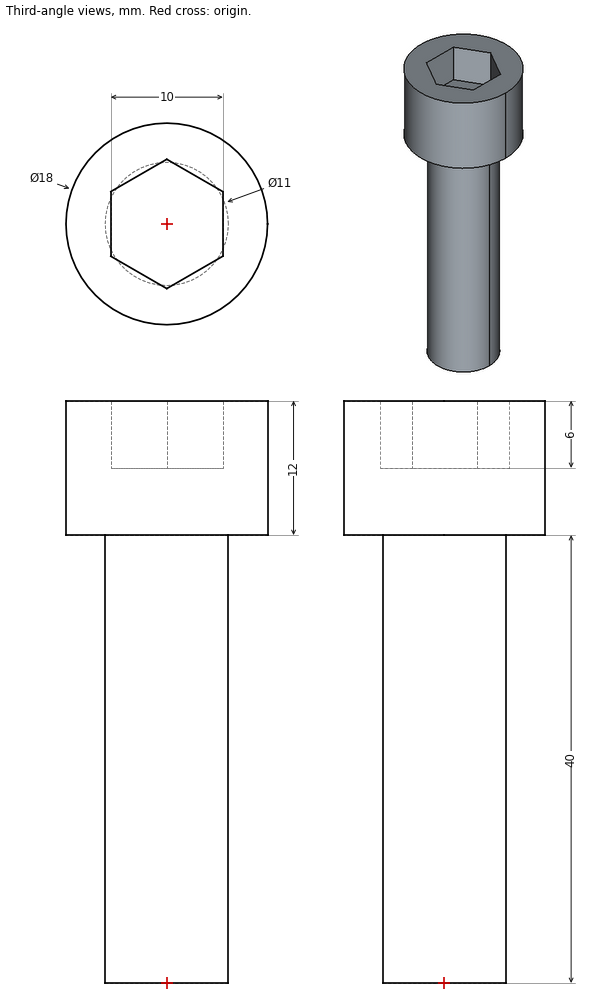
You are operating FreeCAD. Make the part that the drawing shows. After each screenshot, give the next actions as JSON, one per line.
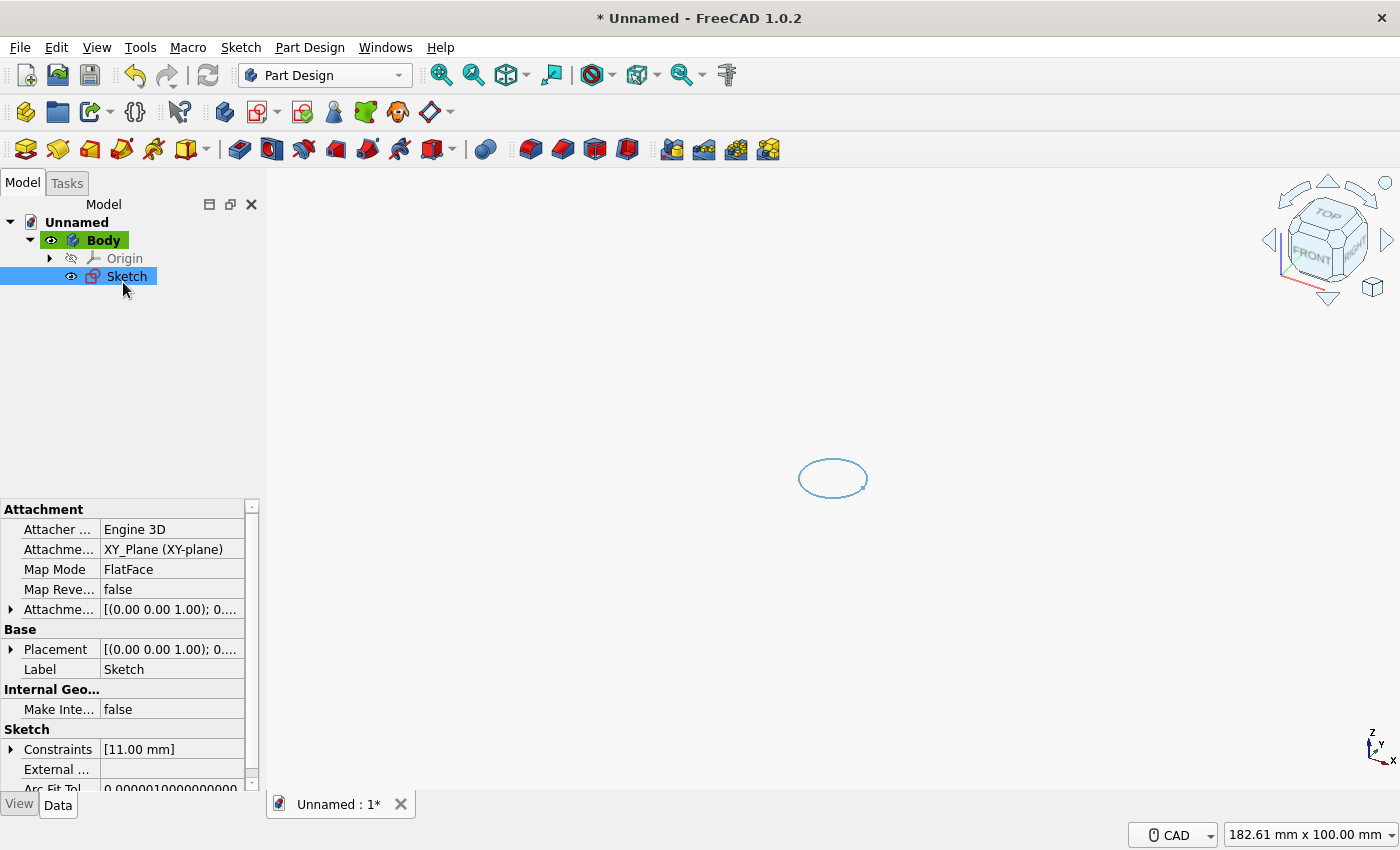
{"action": "left_click", "coordinate": [26, 150]}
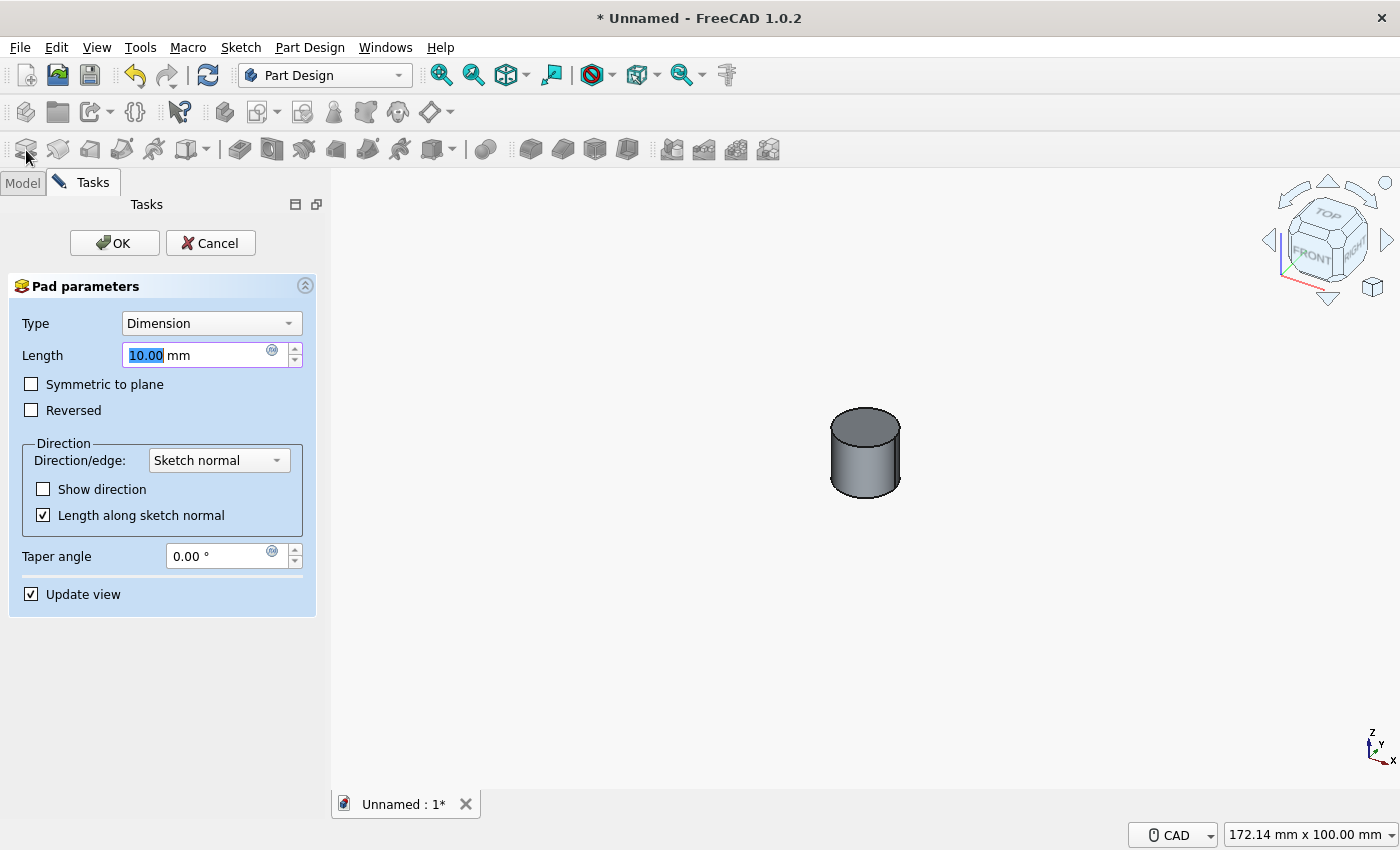
{"action": "type", "text": "40"}
{"action": "key", "text": "Tab"}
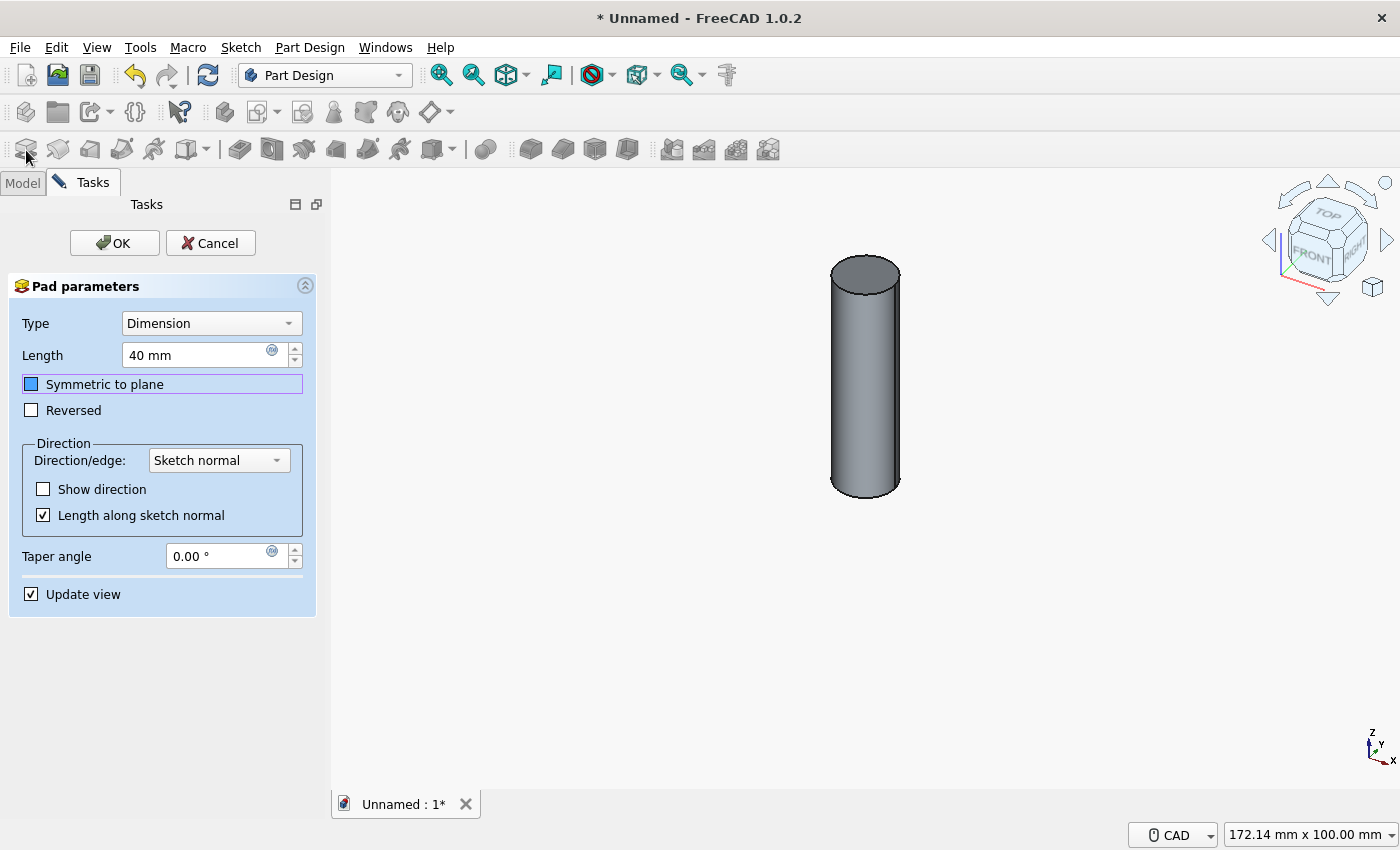
{"action": "left_click", "coordinate": [115, 243]}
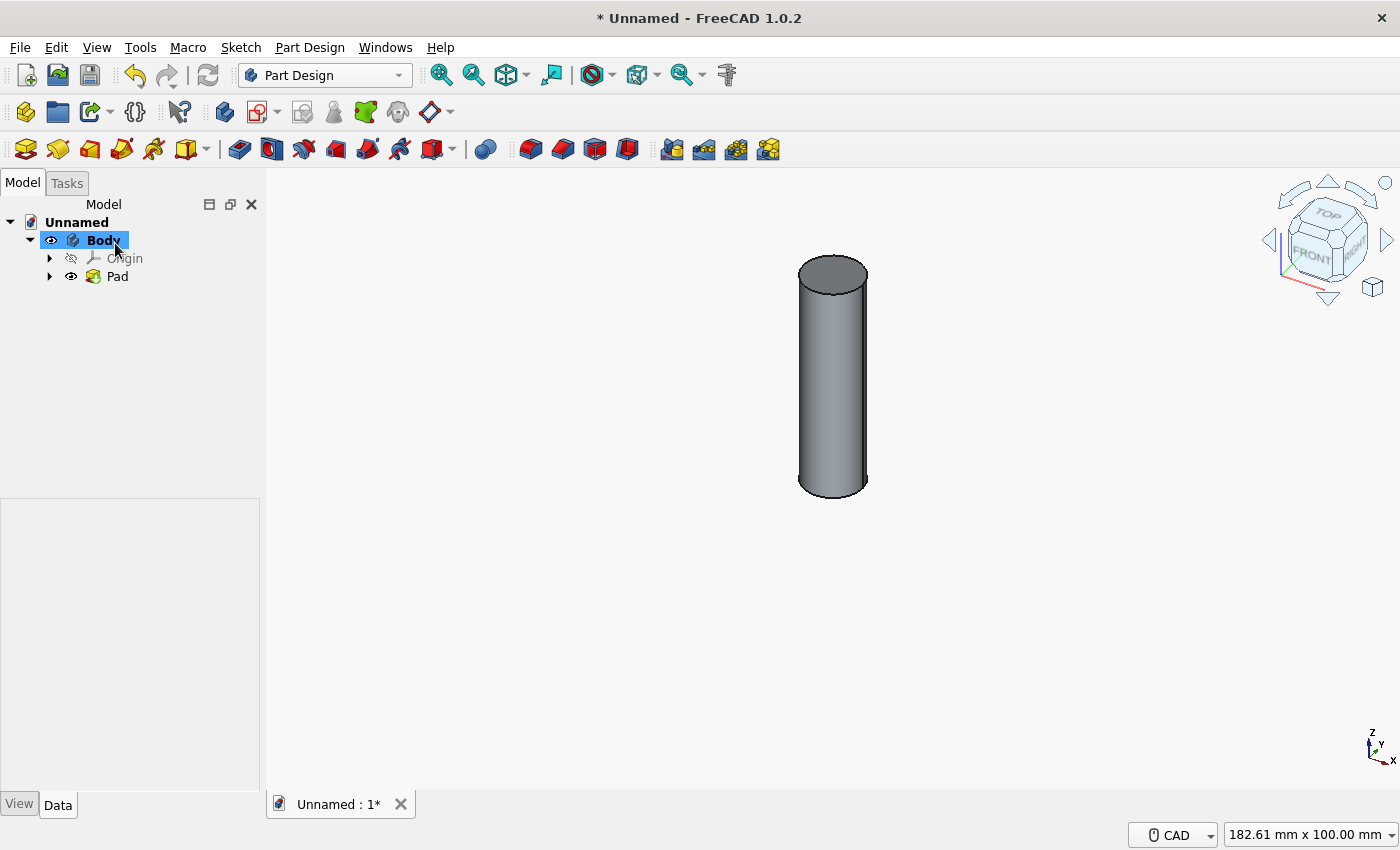
{"action": "left_click", "coordinate": [442, 76]}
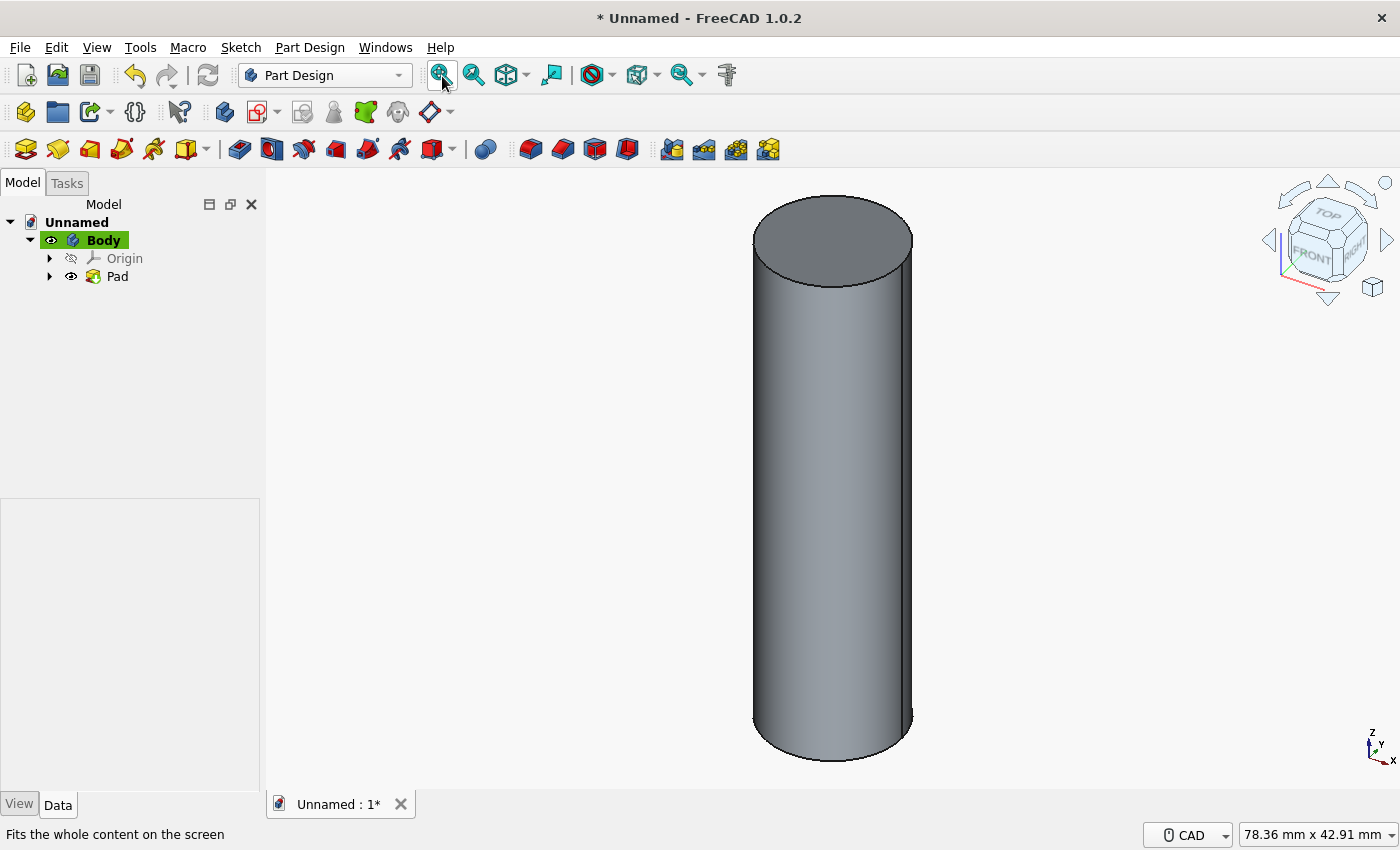
{"action": "left_click", "coordinate": [833, 240]}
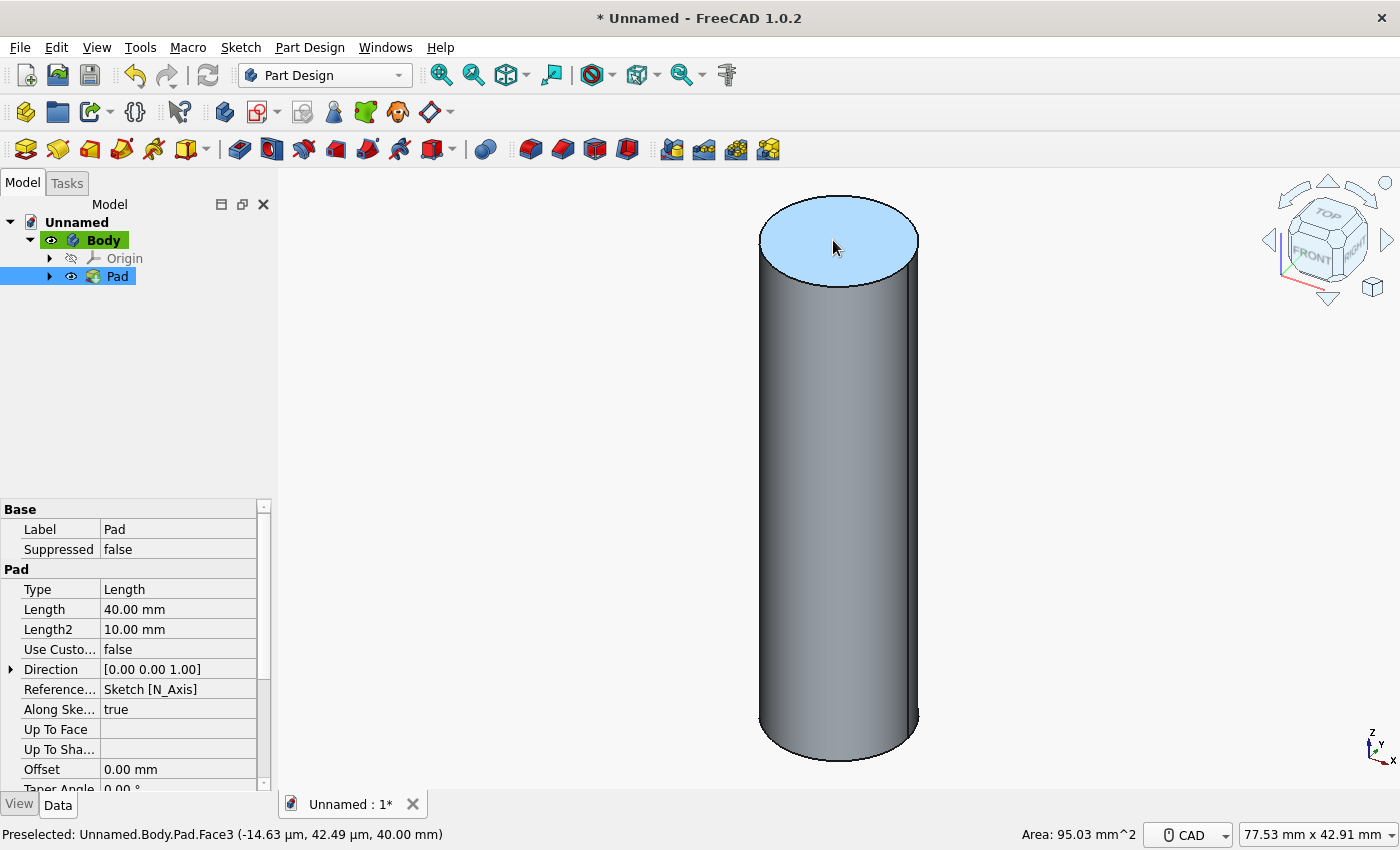
{"action": "left_click", "coordinate": [258, 112]}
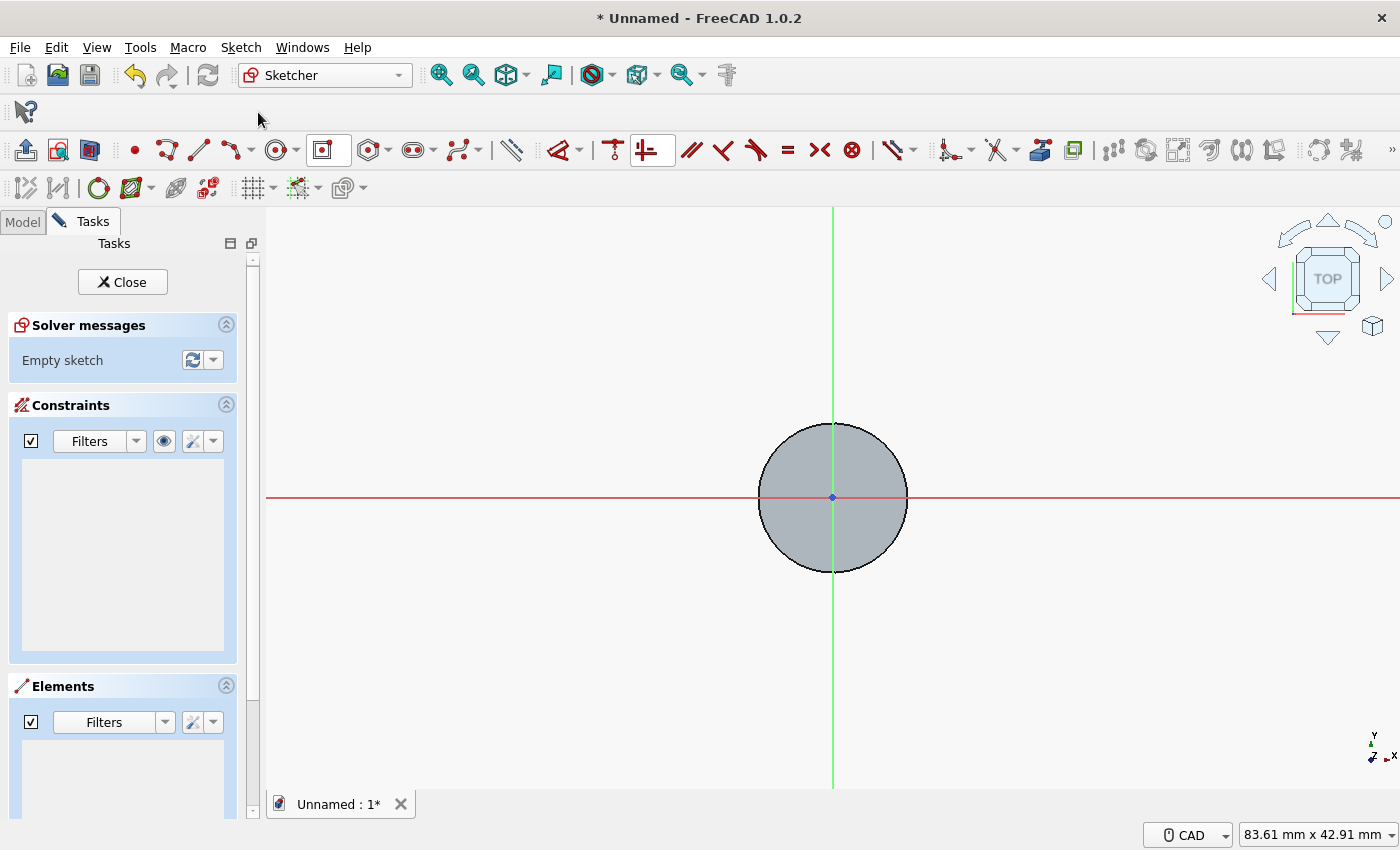
{"action": "scroll", "coordinate": [972, 498], "scroll_direction": "up", "scroll_amount": 2}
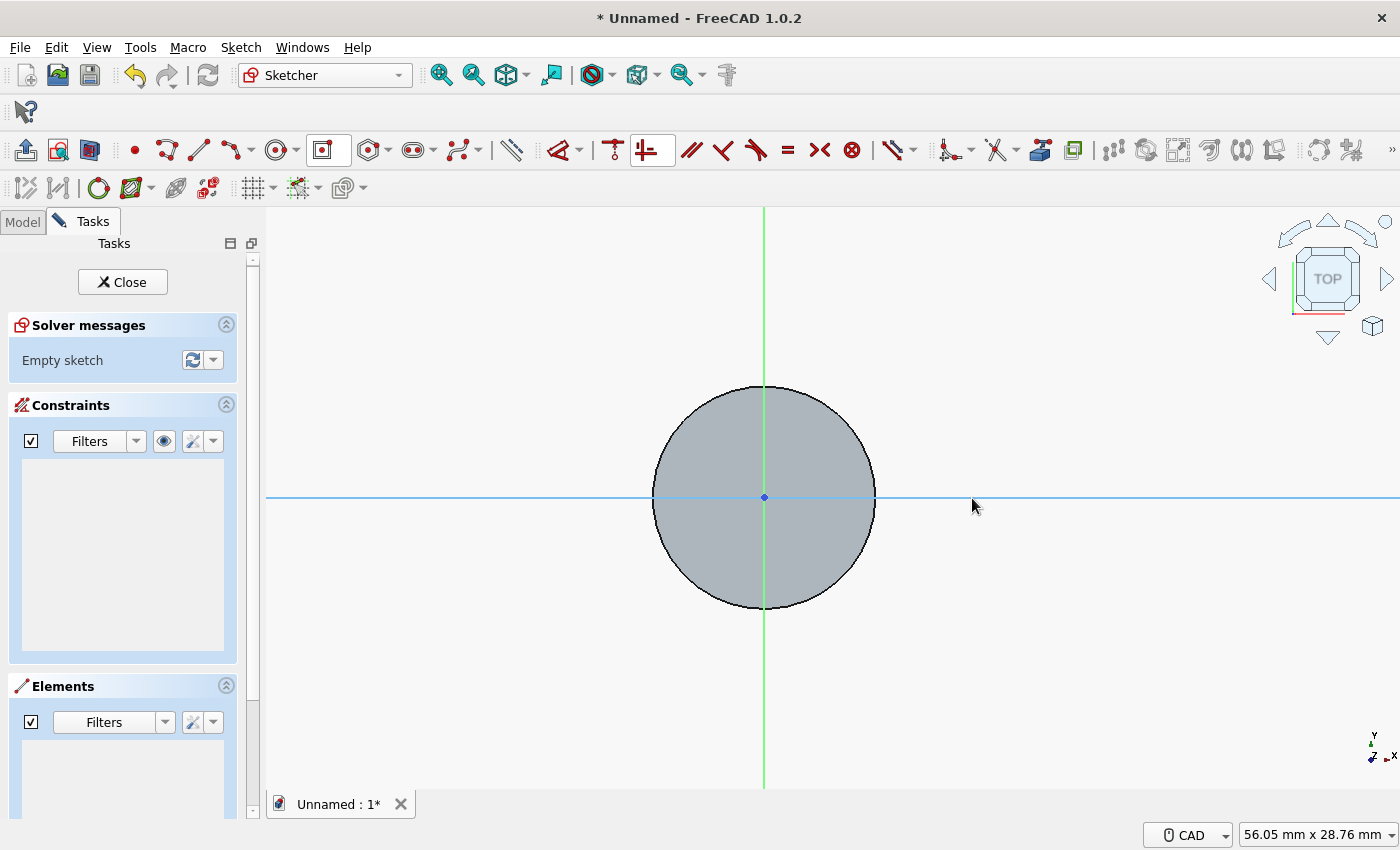
{"action": "key", "text": "g c"}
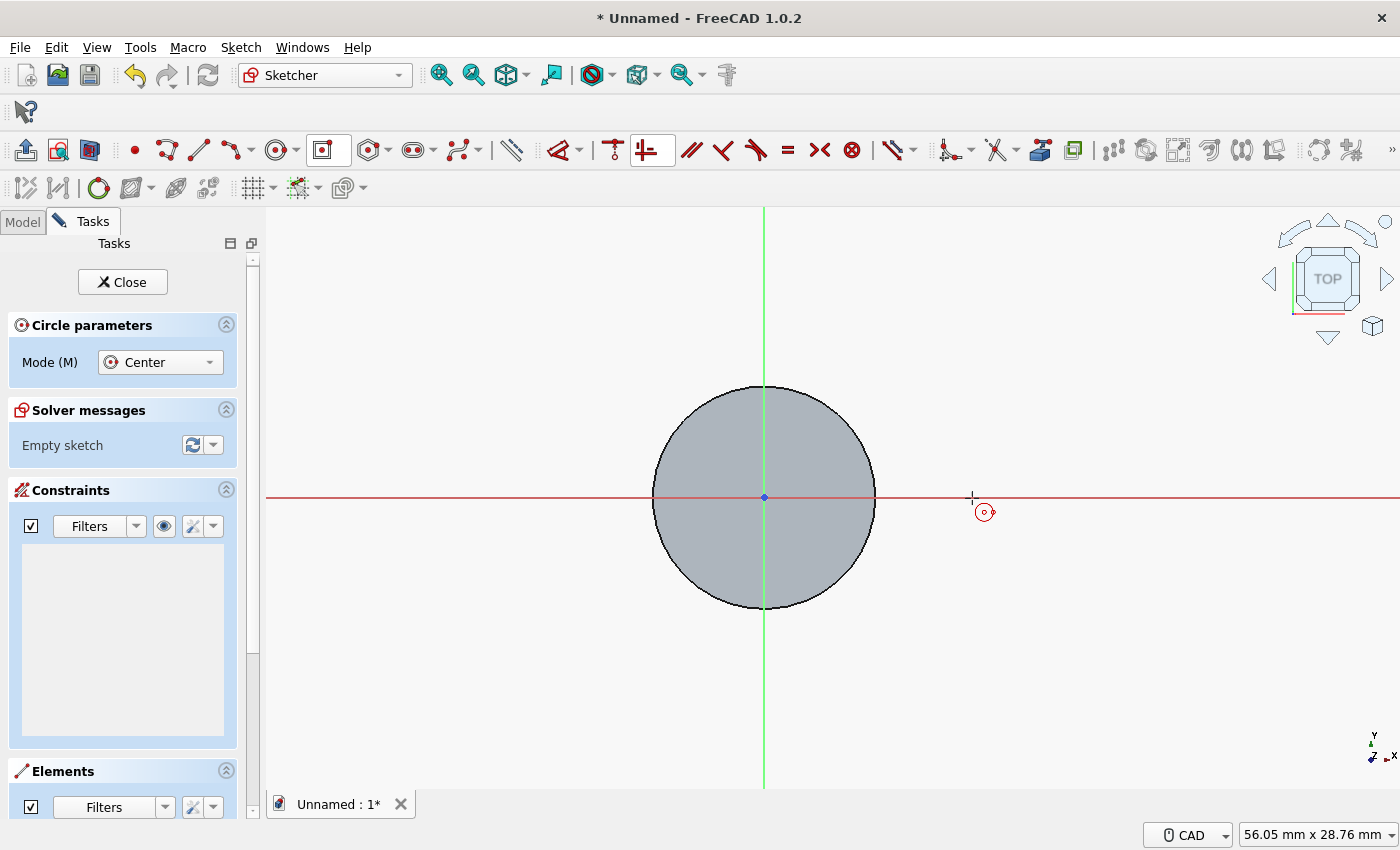
{"action": "left_click", "coordinate": [764, 498]}
{"action": "mouse_move", "coordinate": [893, 369]}